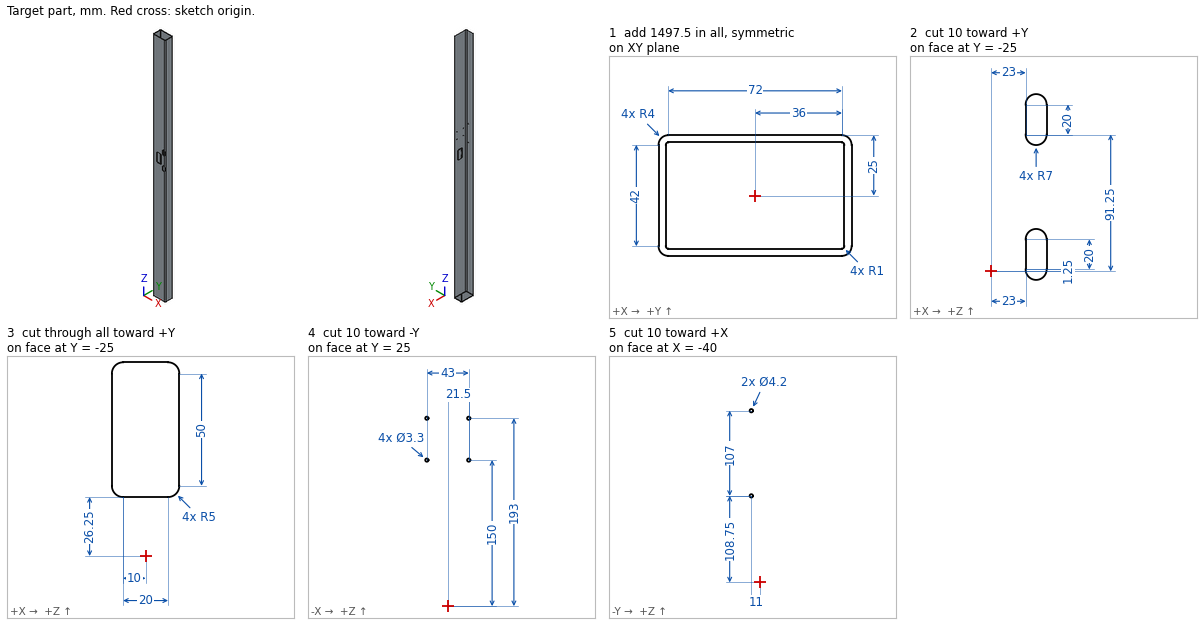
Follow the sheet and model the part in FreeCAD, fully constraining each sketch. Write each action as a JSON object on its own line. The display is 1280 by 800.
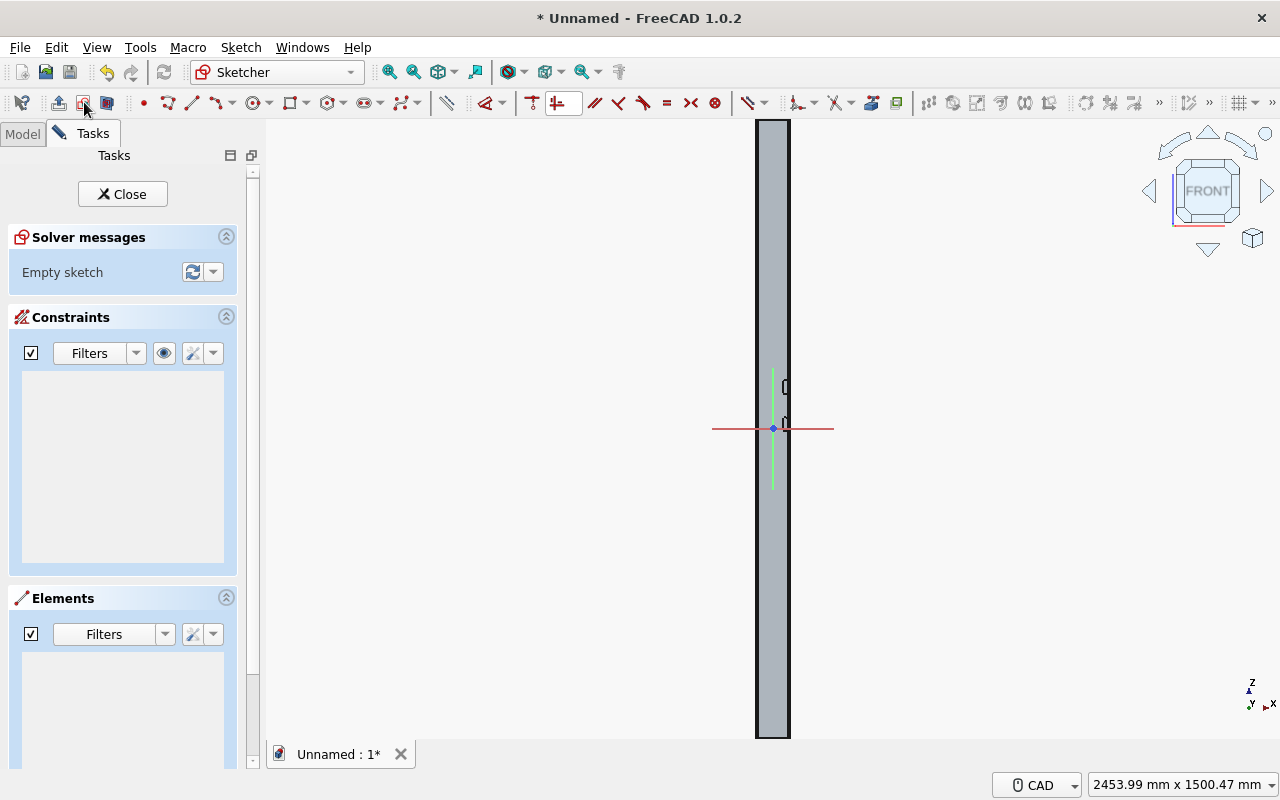
{"action": "scroll", "coordinate": [780, 409], "scroll_direction": "up", "scroll_amount": 12}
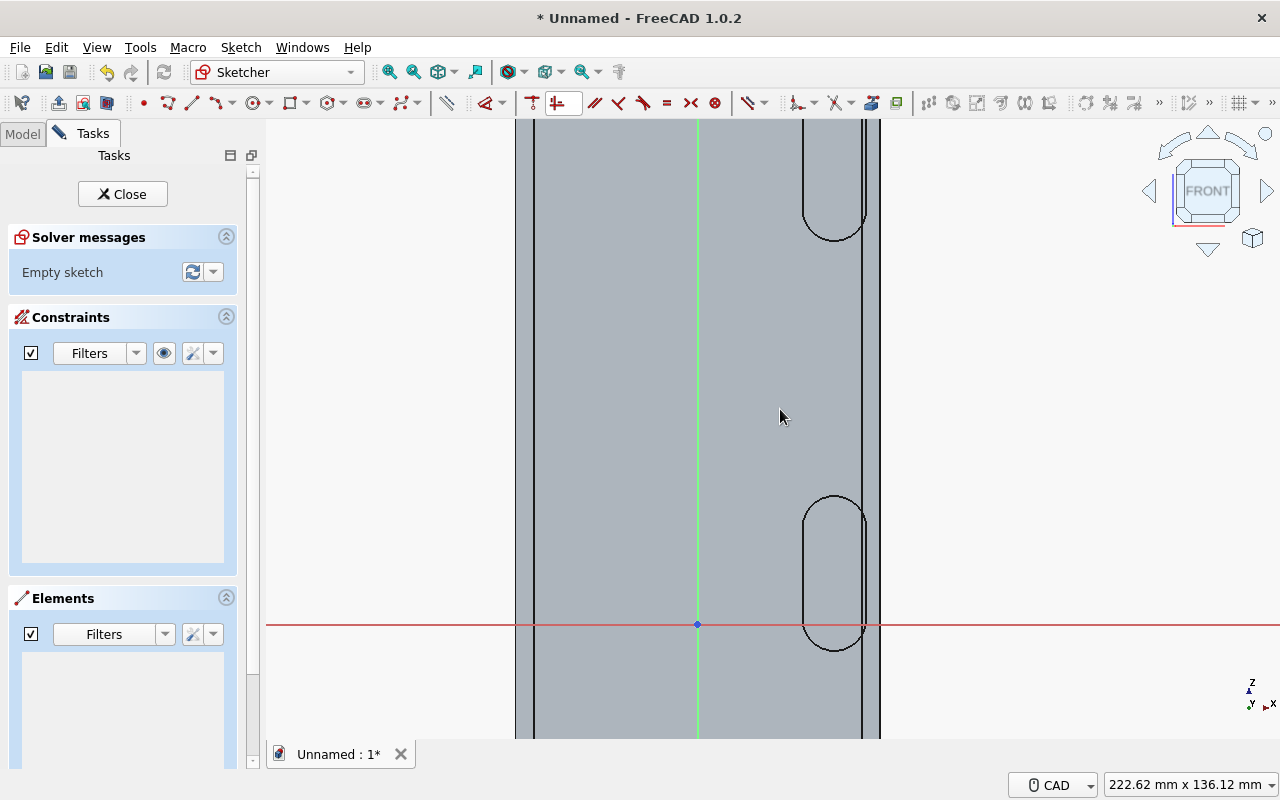
{"action": "key", "text": "g l"}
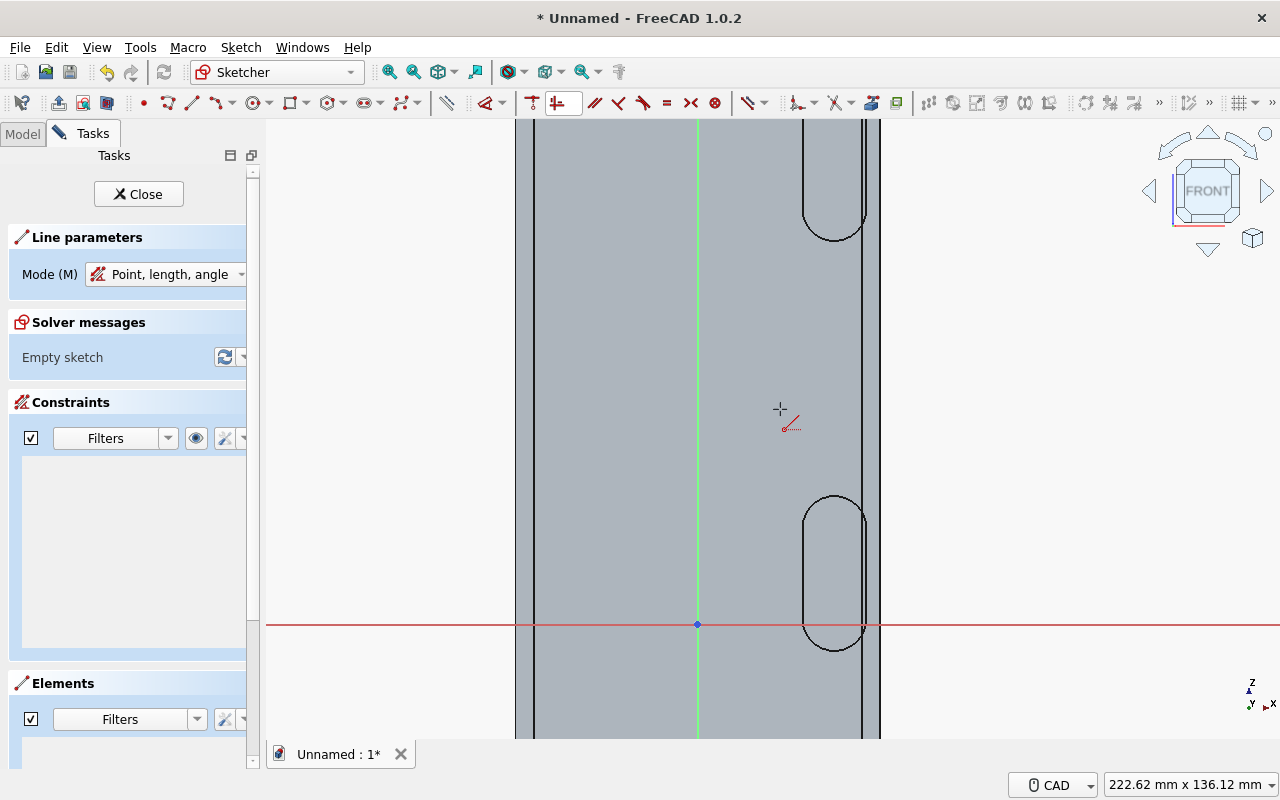
{"action": "left_click", "coordinate": [652, 505]}
{"action": "left_click", "coordinate": [743, 505]}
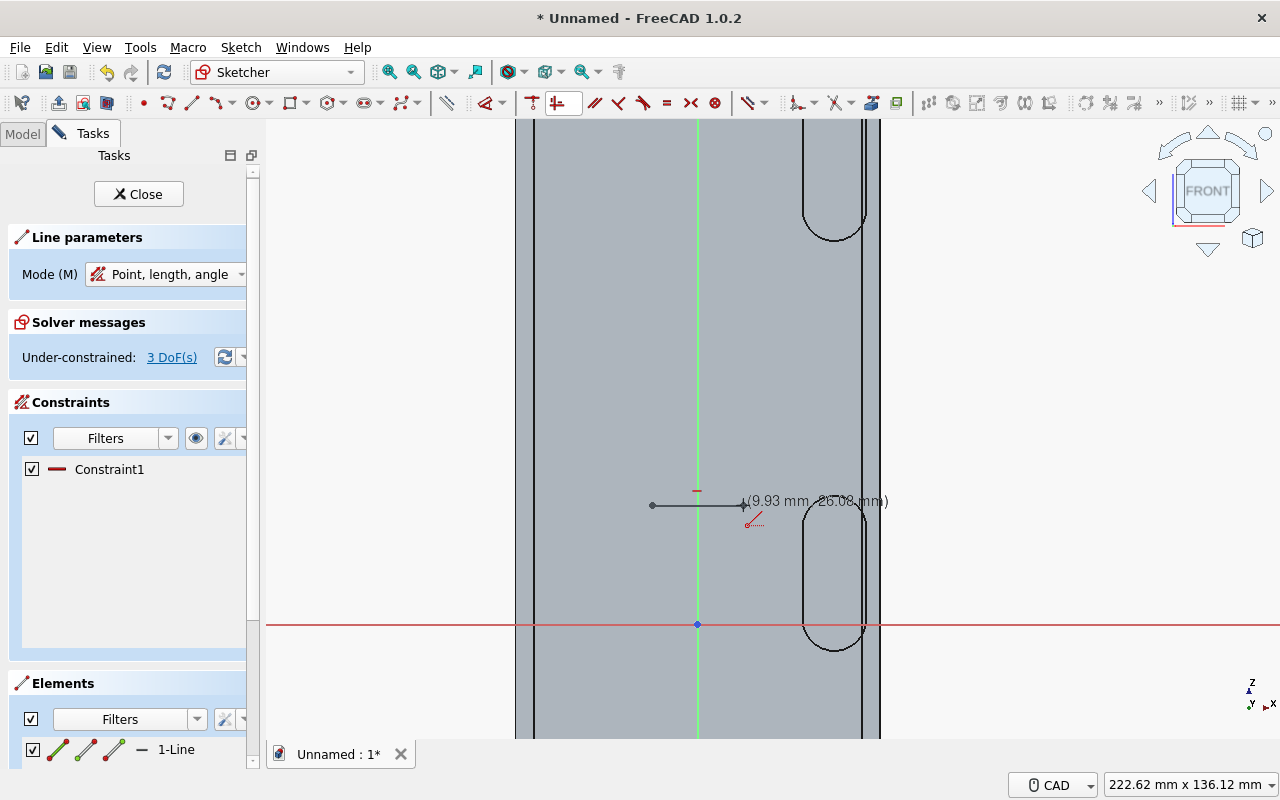
{"action": "left_click", "coordinate": [766, 482]}
{"action": "left_click", "coordinate": [766, 255]}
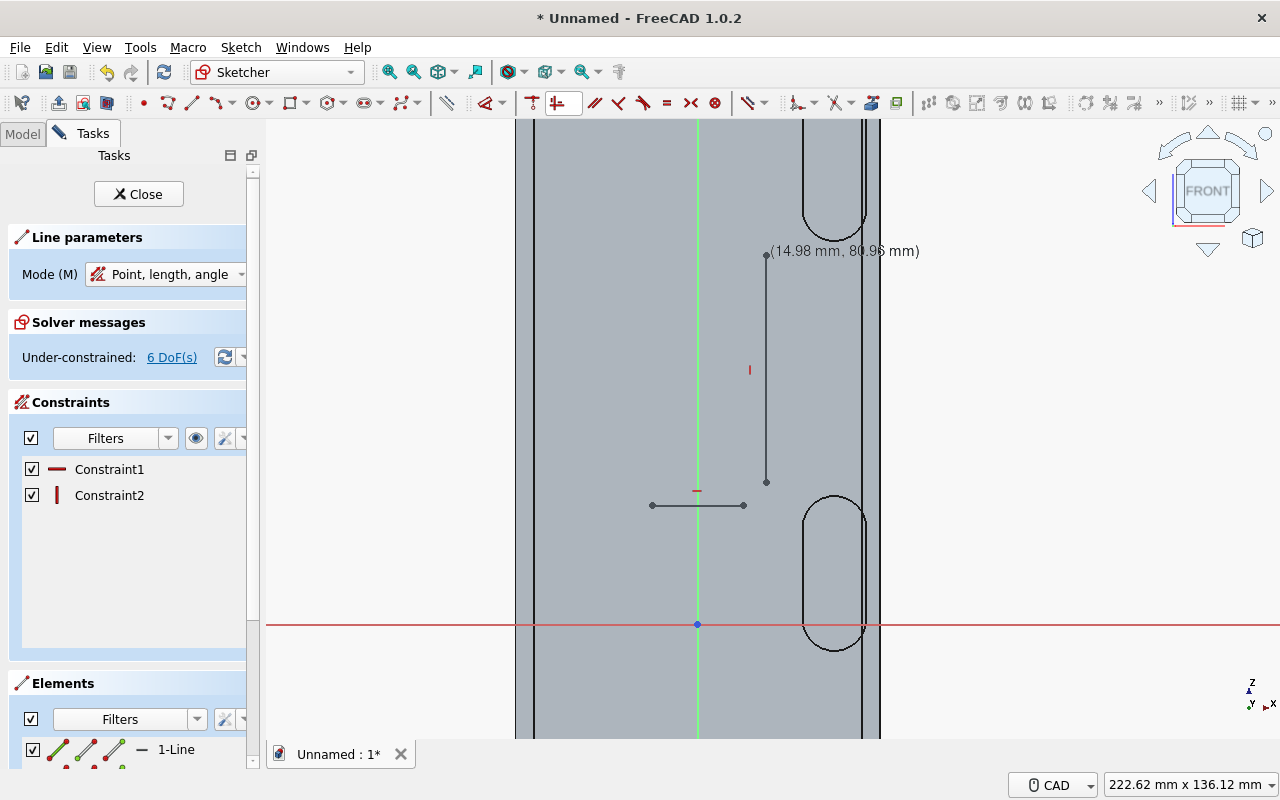
{"action": "left_click", "coordinate": [743, 232]}
{"action": "left_click", "coordinate": [652, 232]}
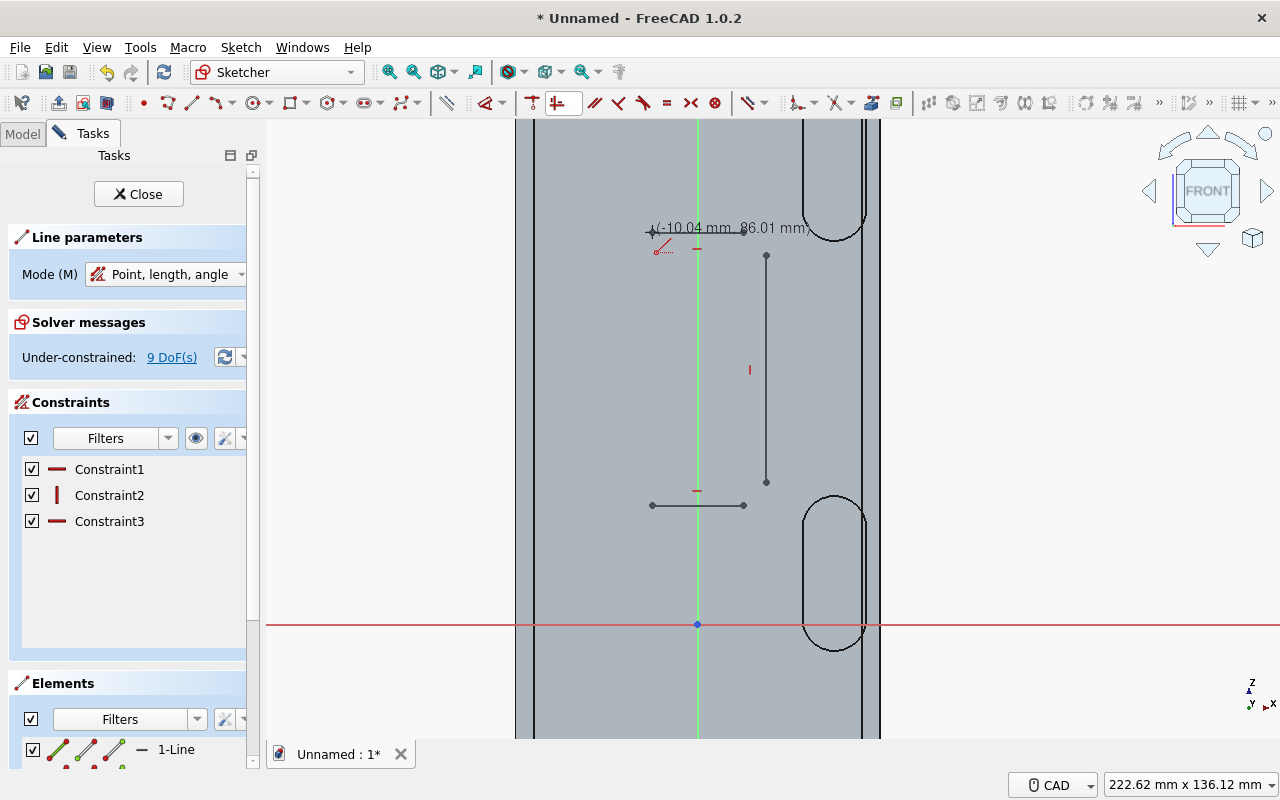
{"action": "left_click", "coordinate": [629, 255]}
{"action": "left_click", "coordinate": [629, 482]}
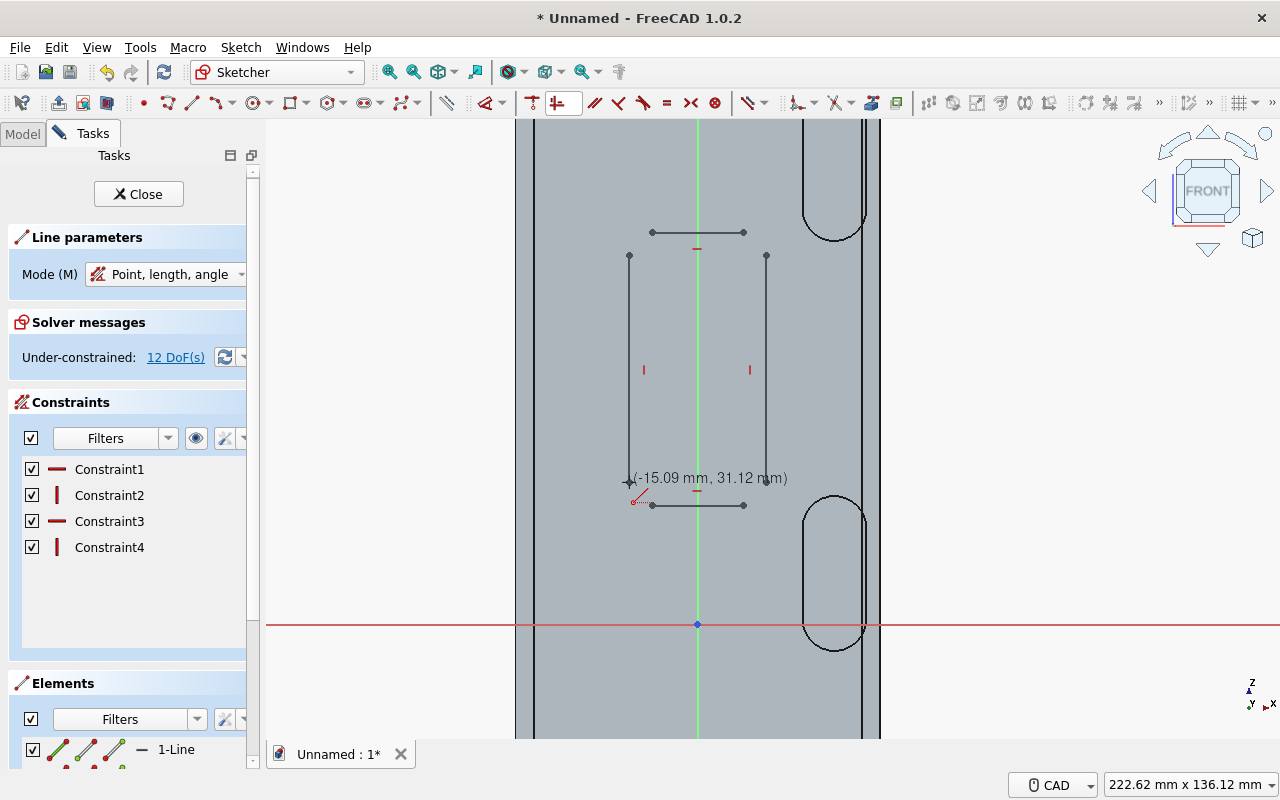
{"action": "key", "text": "g 3 a"}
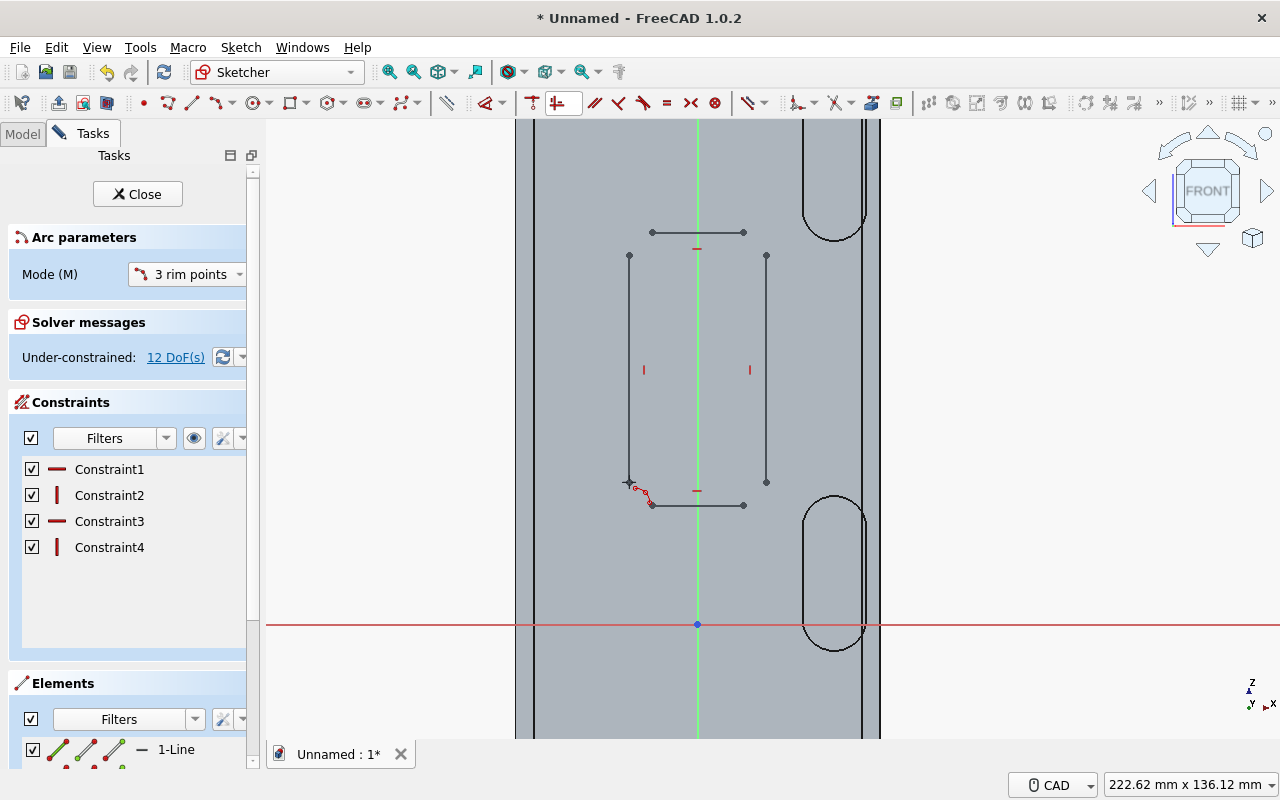
{"action": "left_click", "coordinate": [743, 506]}
{"action": "left_click", "coordinate": [766, 483]}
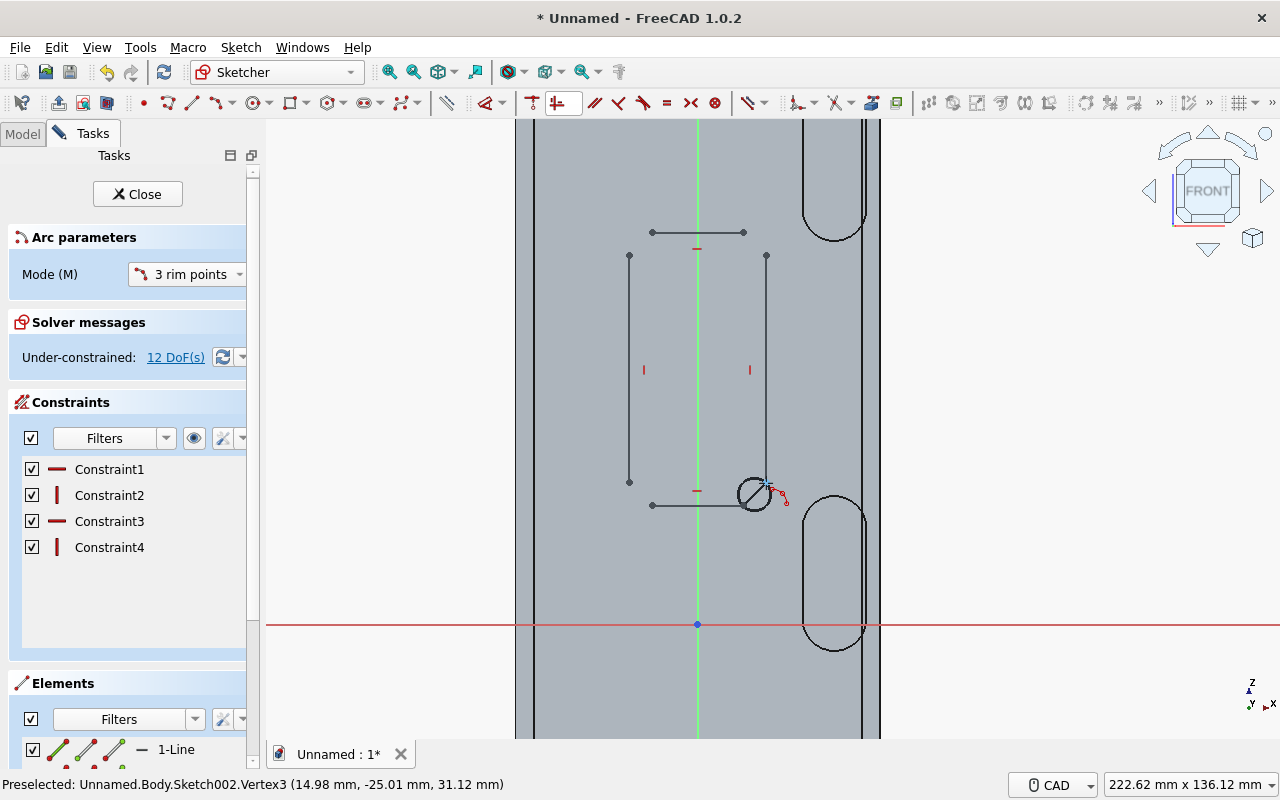
{"action": "scroll", "coordinate": [759, 499], "scroll_direction": "up", "scroll_amount": 5}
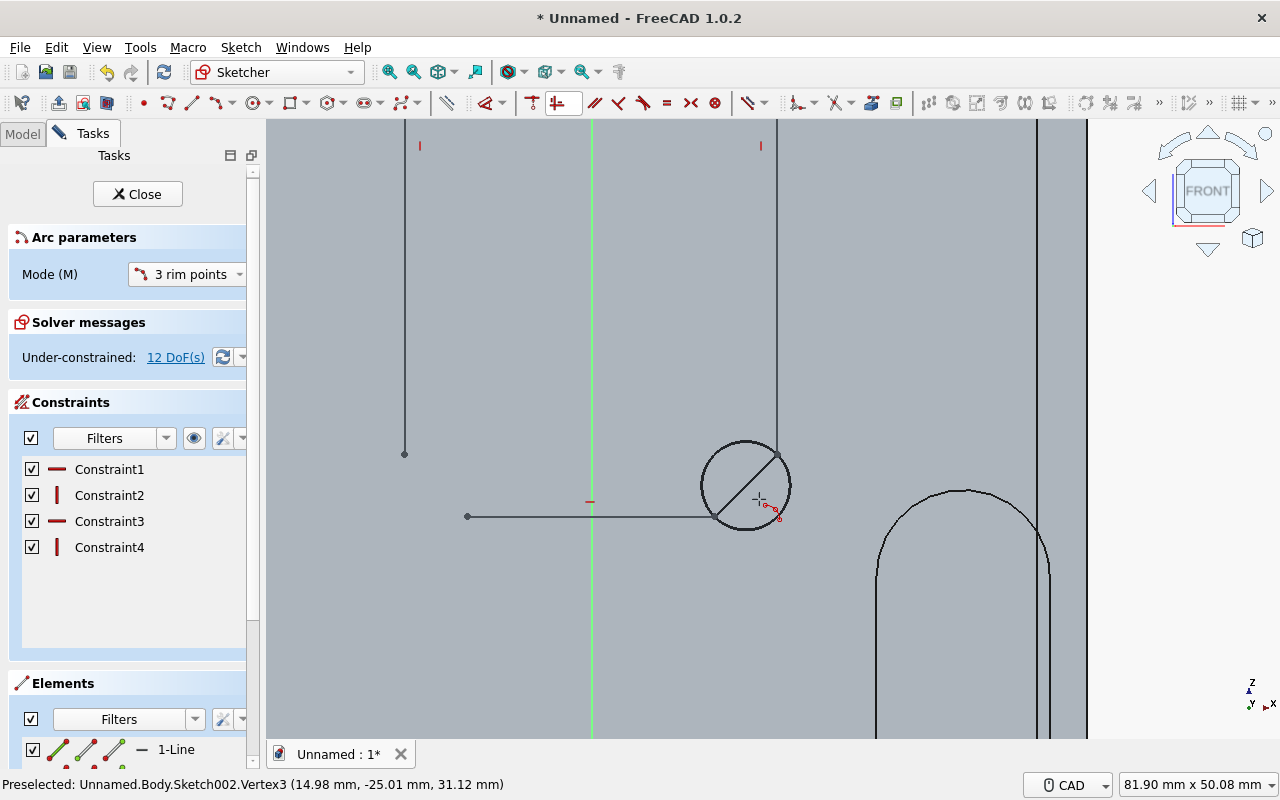
{"action": "left_click", "coordinate": [759, 497]}